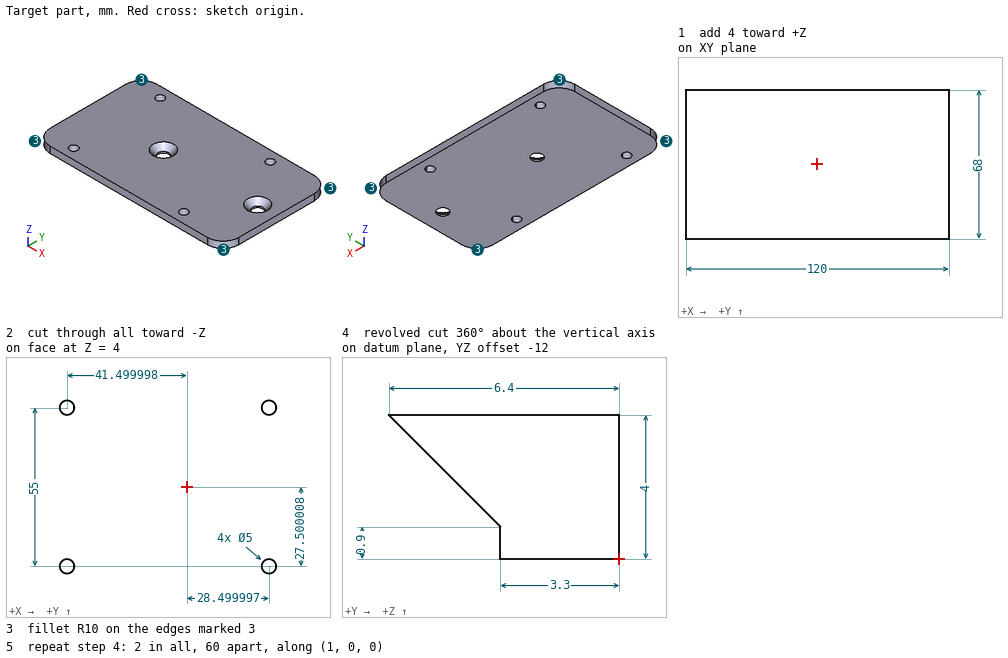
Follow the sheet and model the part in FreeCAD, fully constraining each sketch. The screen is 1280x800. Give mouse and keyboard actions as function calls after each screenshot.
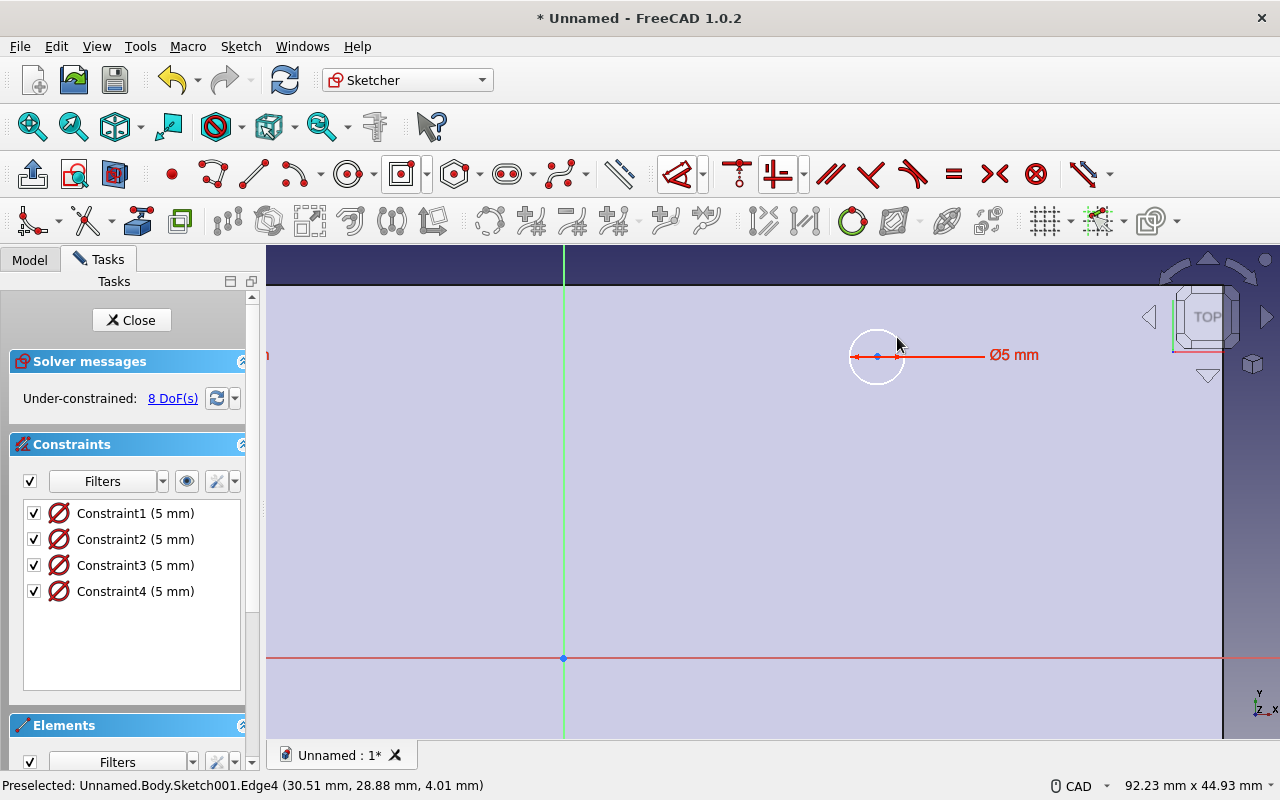
scroll(878, 356, down, 4)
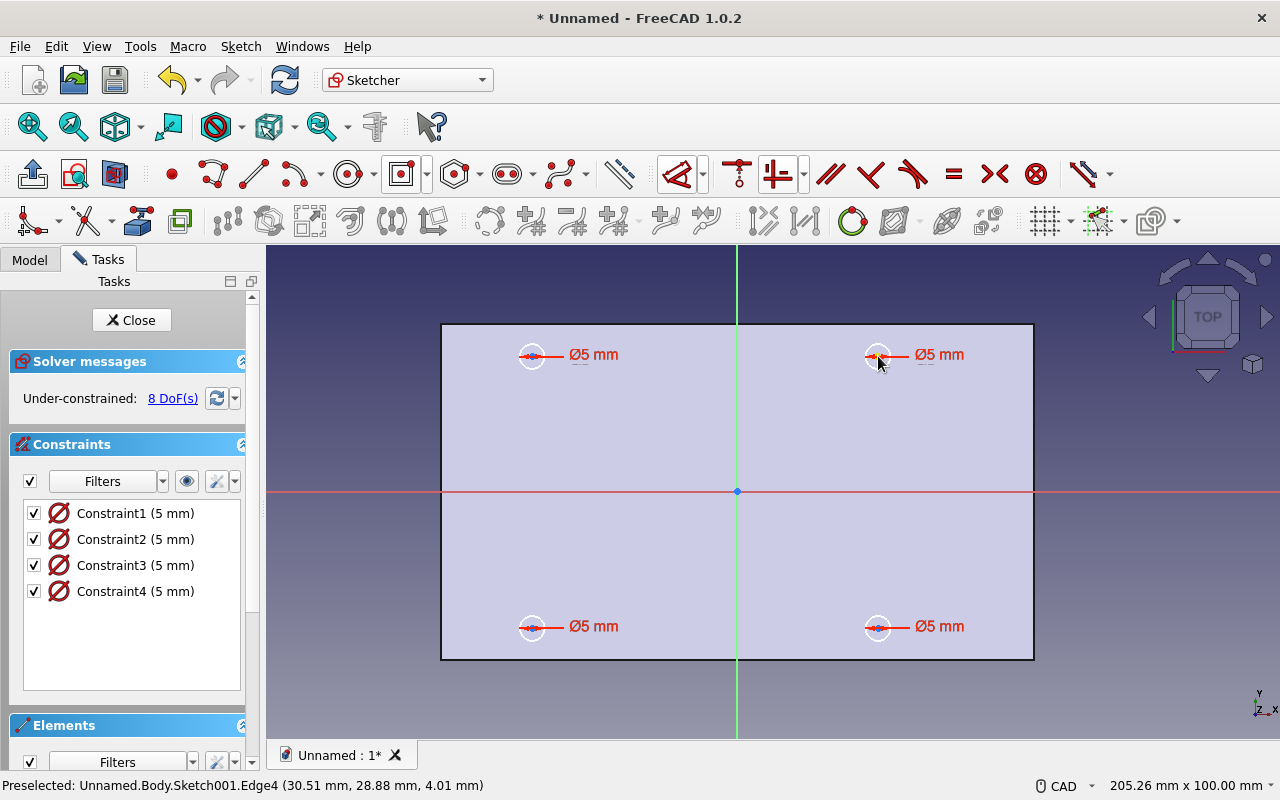
click(532, 357)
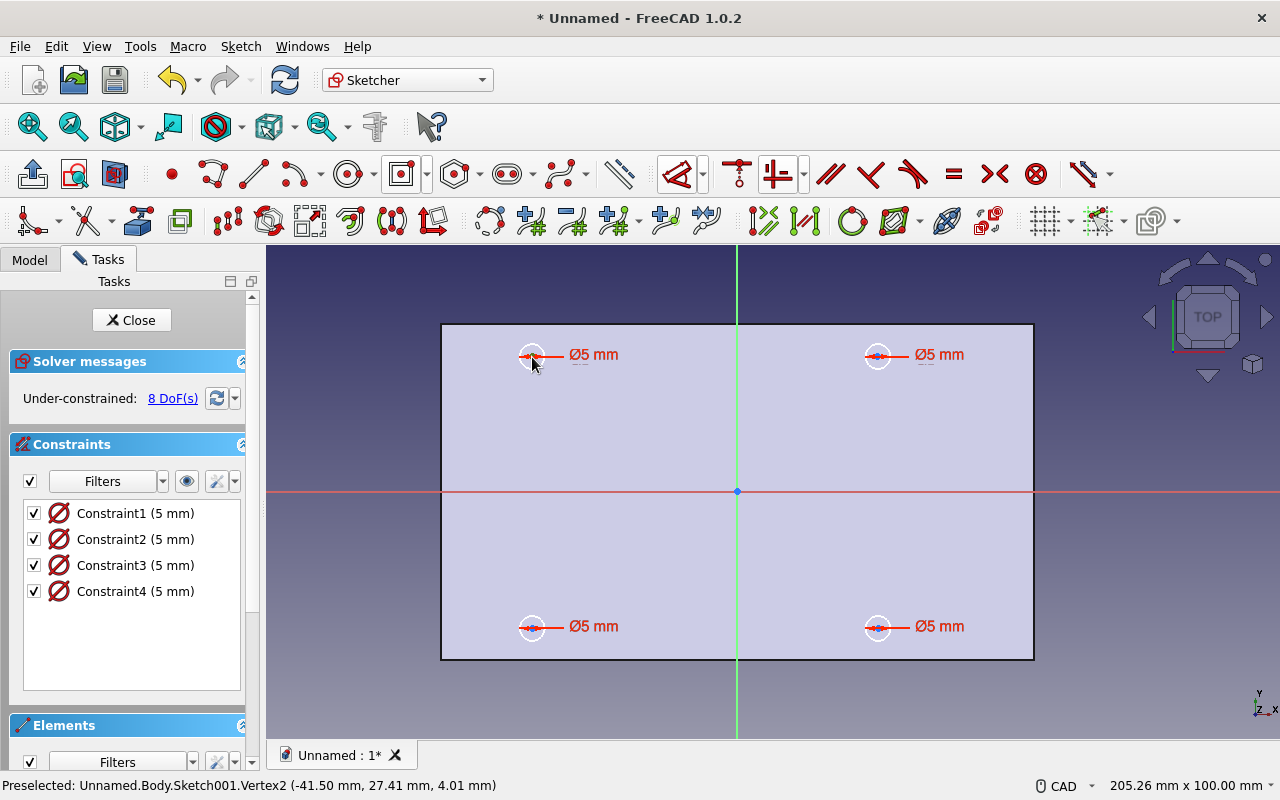
click(532, 628)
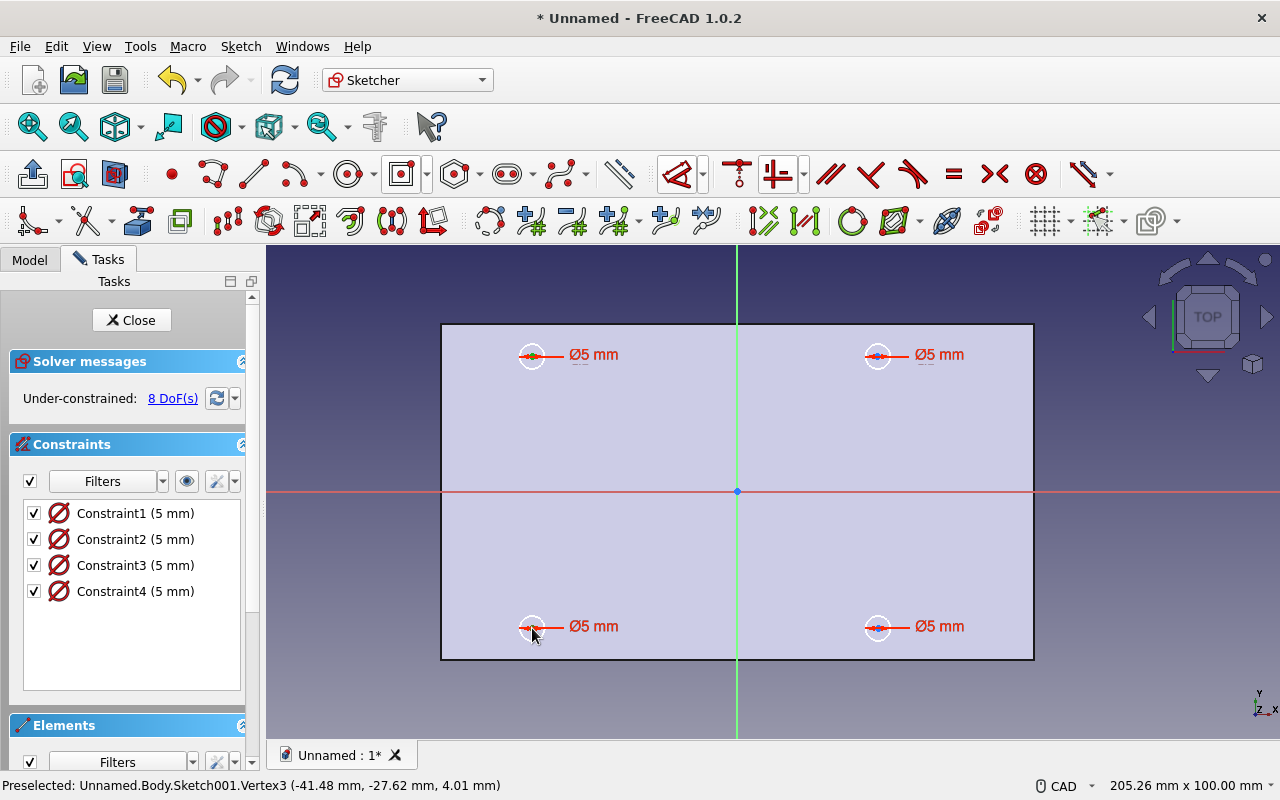
click(804, 174)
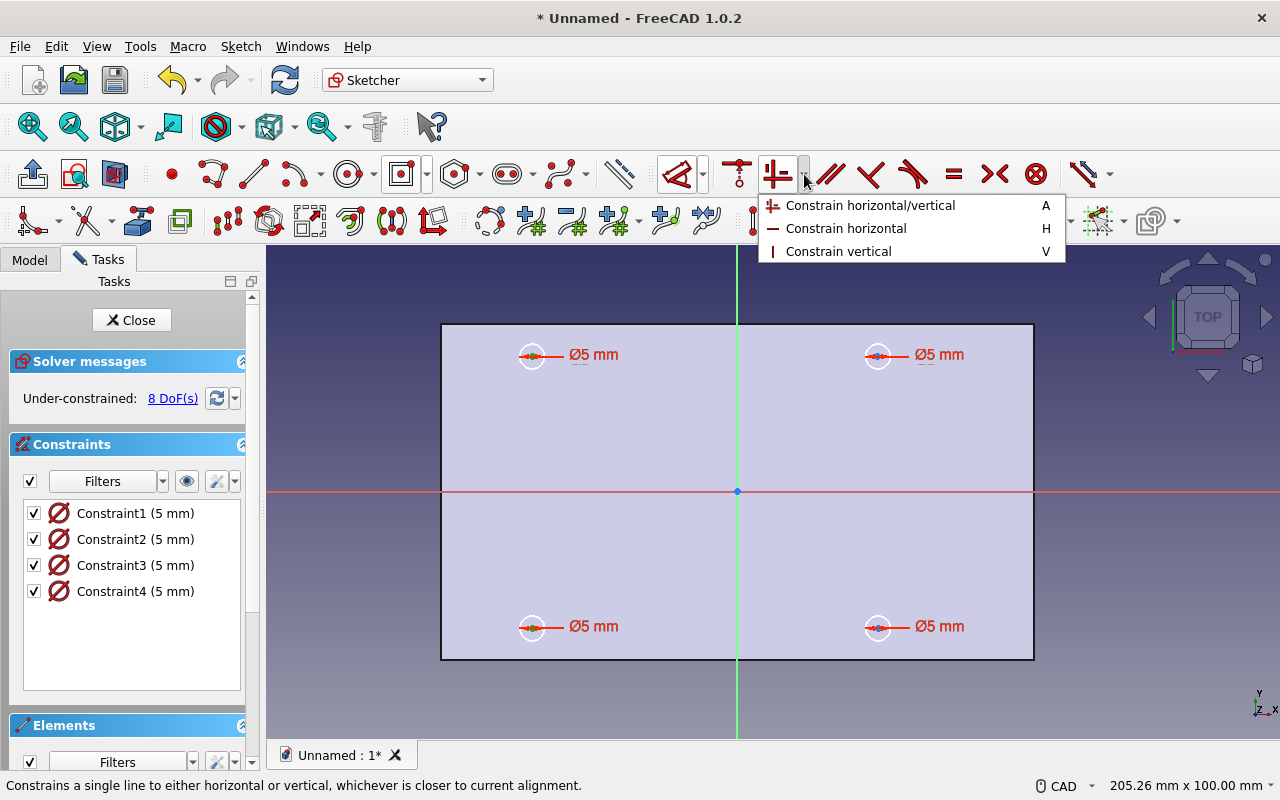
click(912, 252)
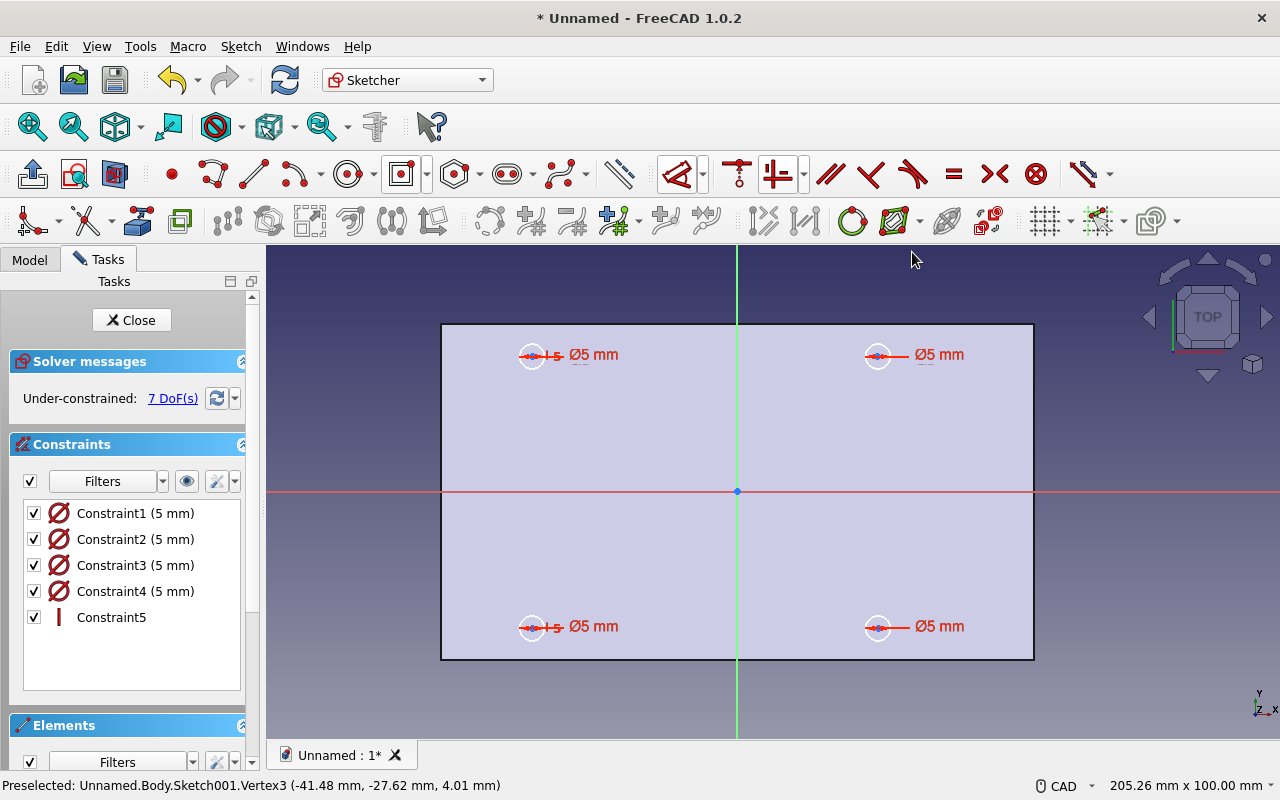
click(878, 628)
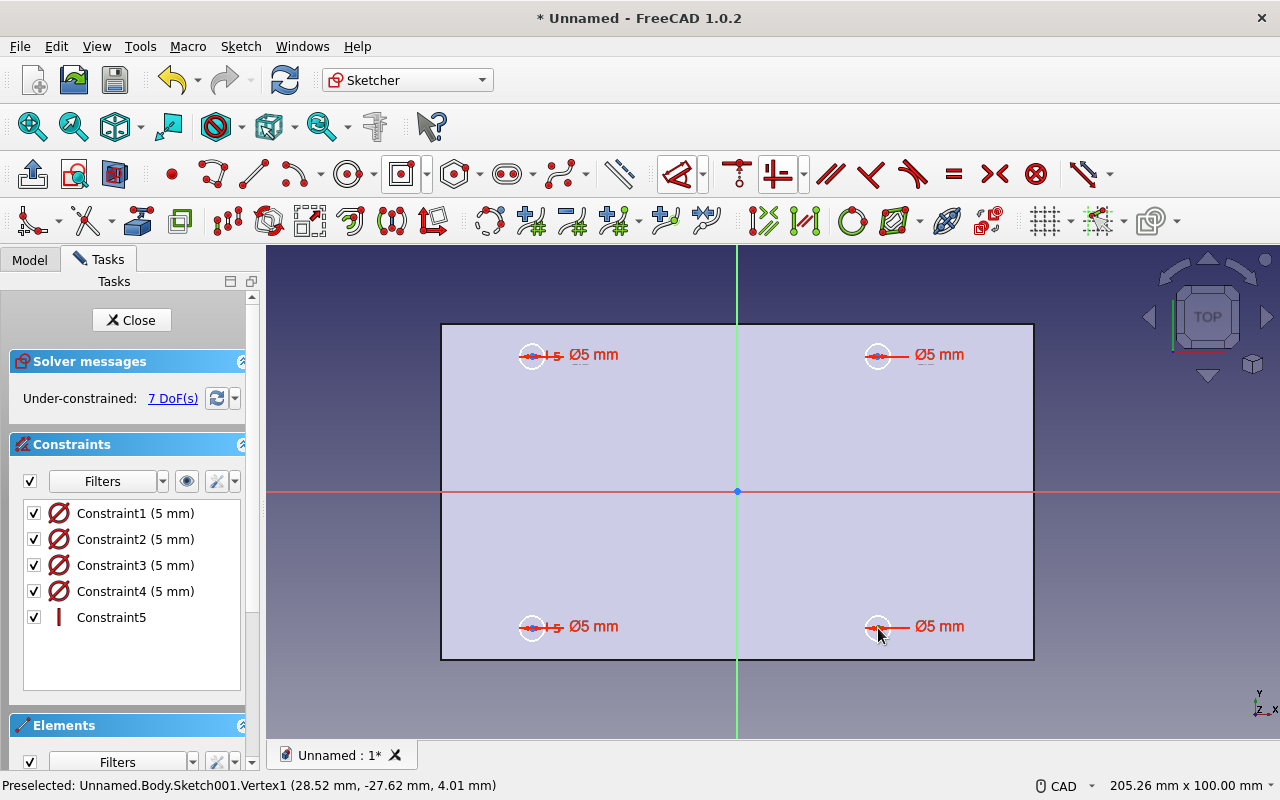
click(532, 628)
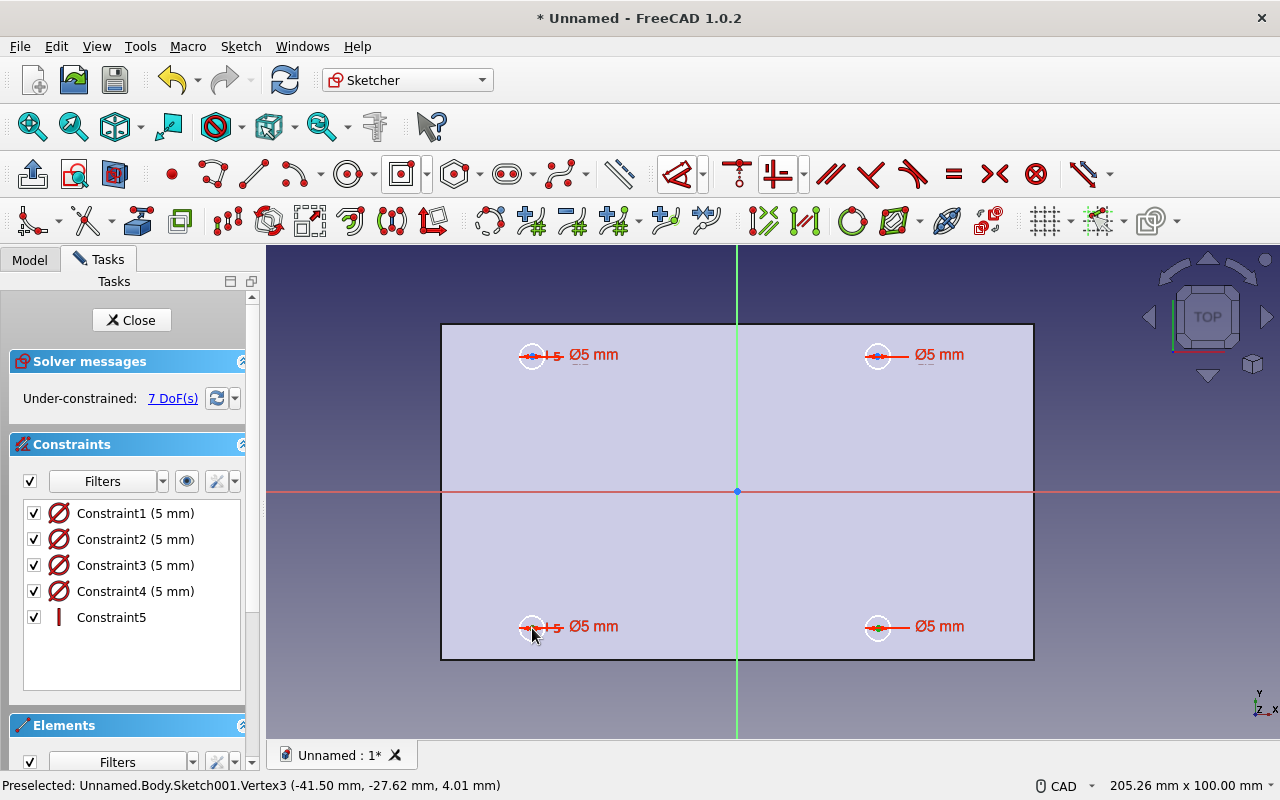
key(h)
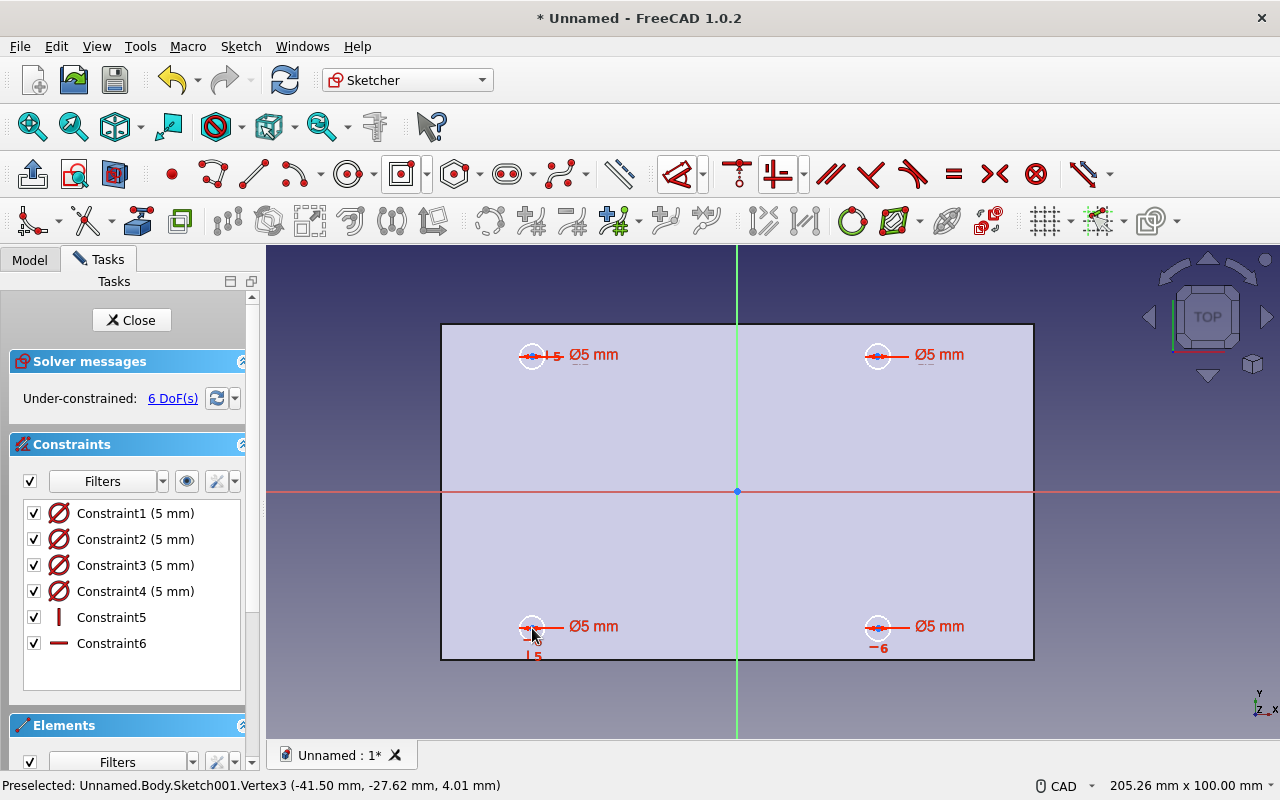
click(878, 628)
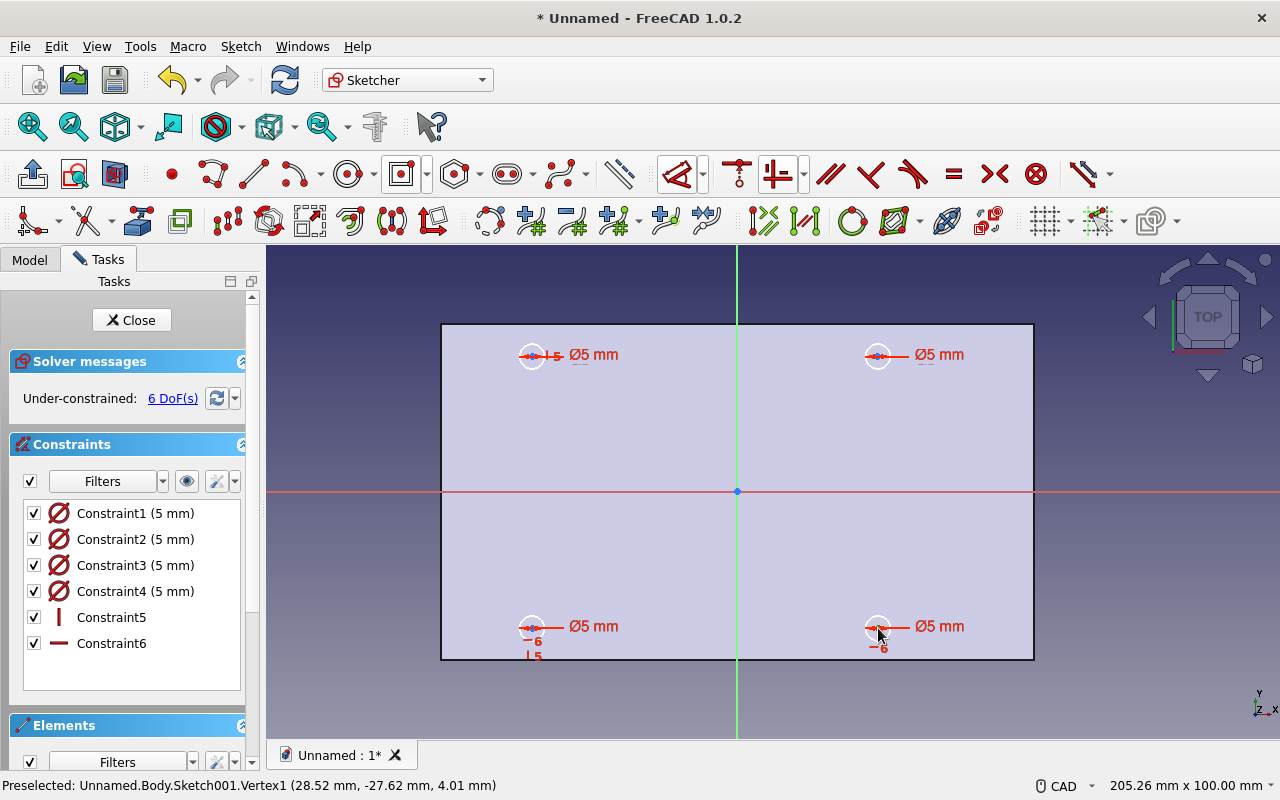
click(878, 357)